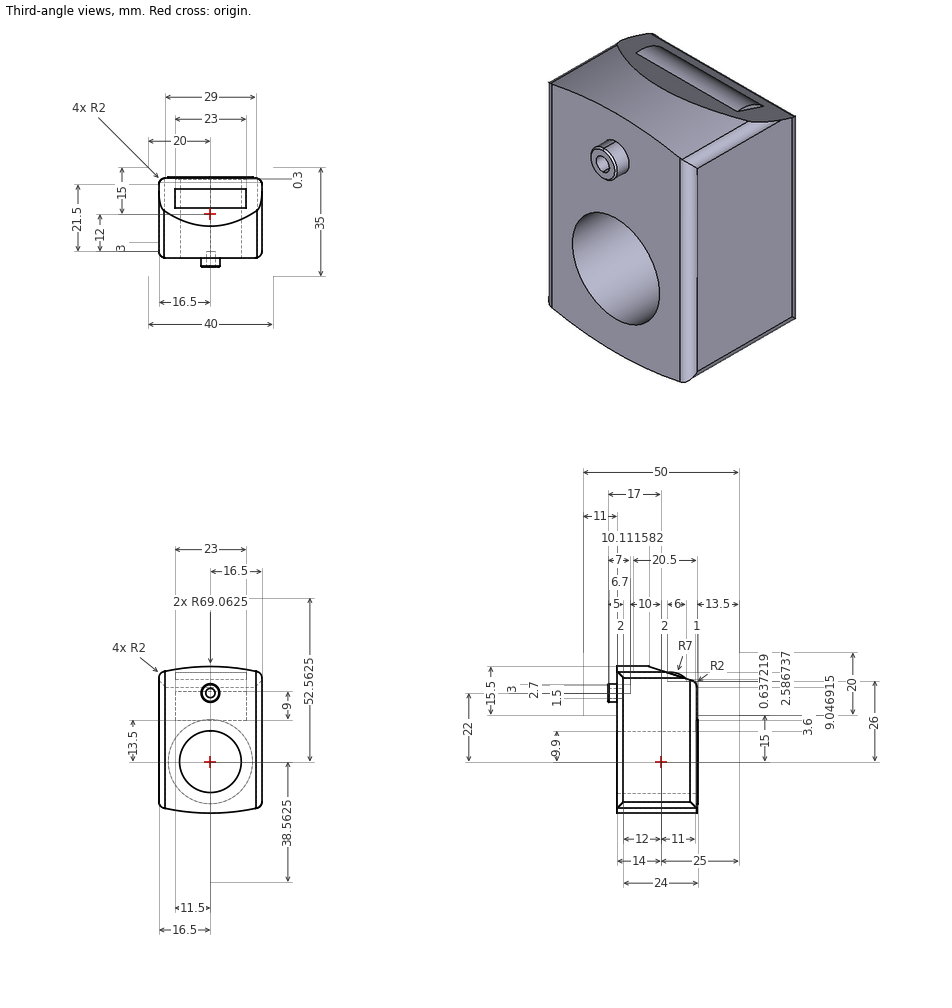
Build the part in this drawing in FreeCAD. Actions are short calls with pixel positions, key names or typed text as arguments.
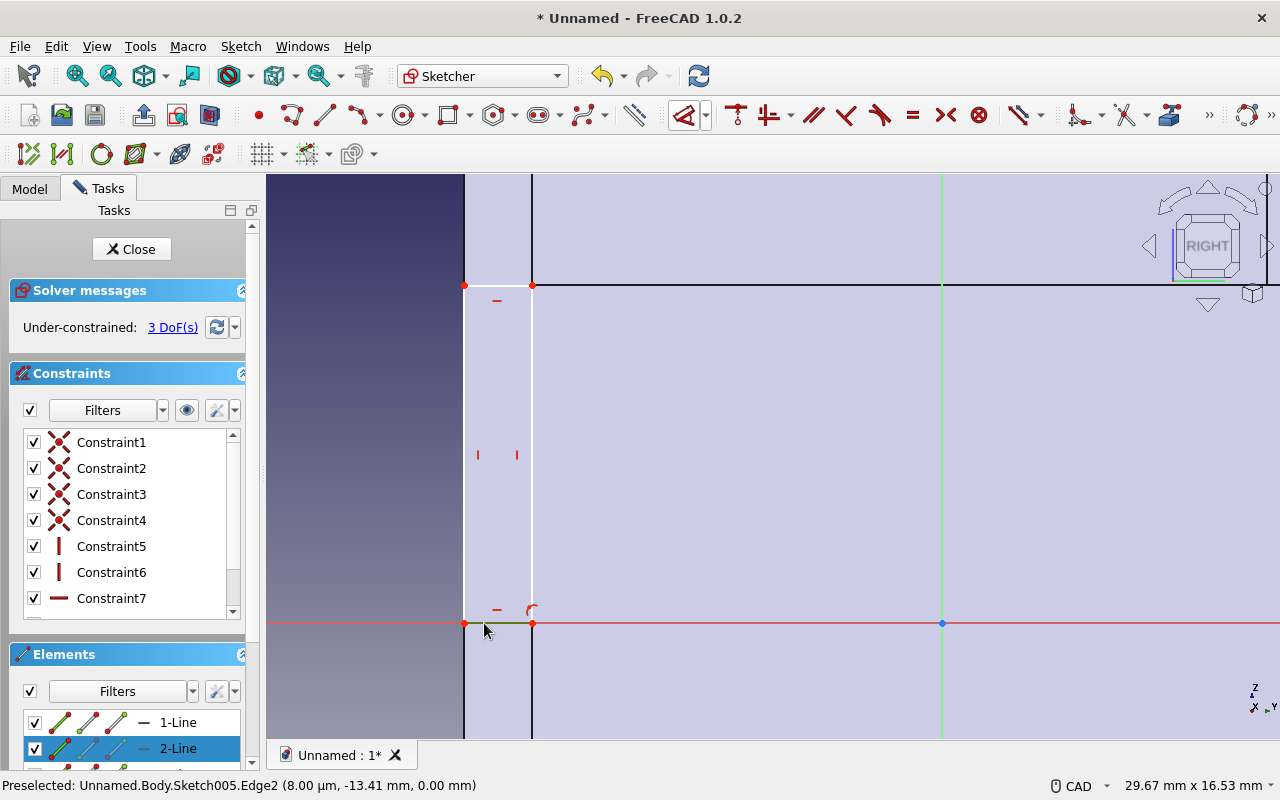
key(l)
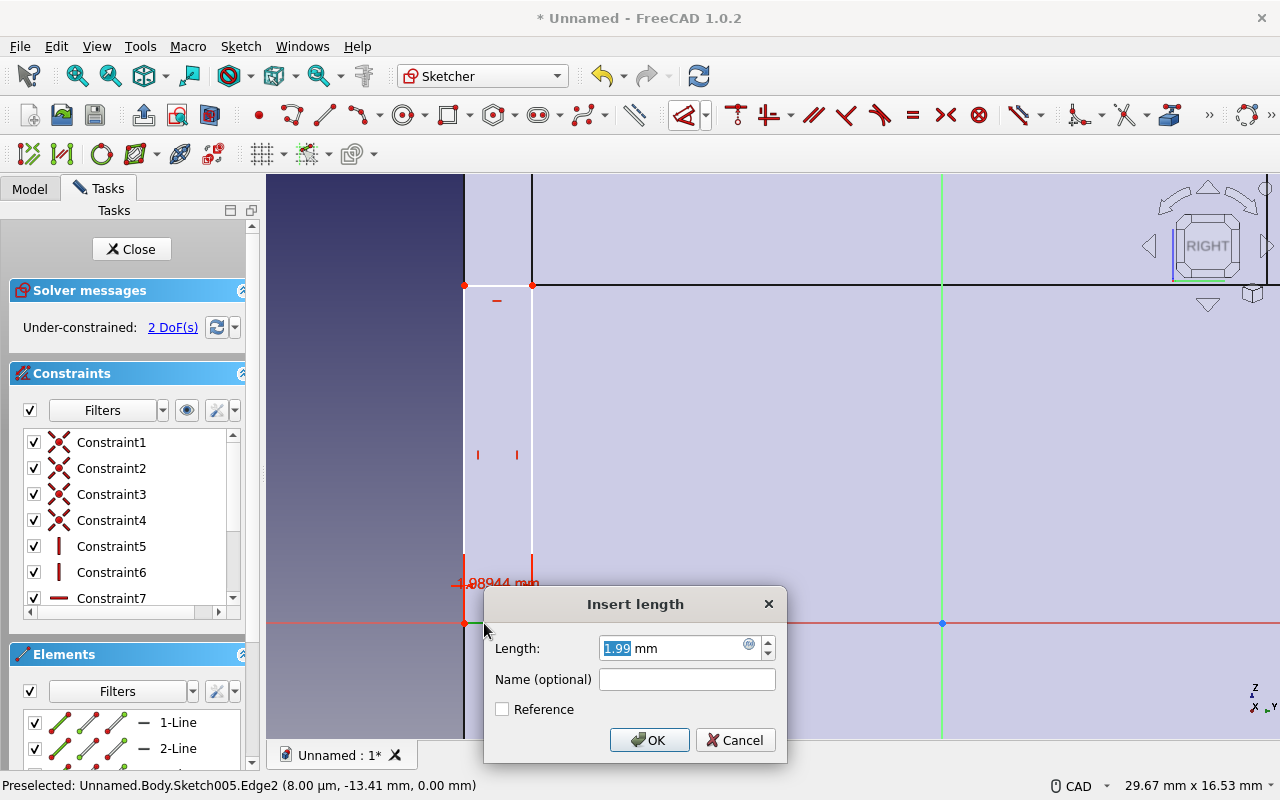
text(2)
key(Return)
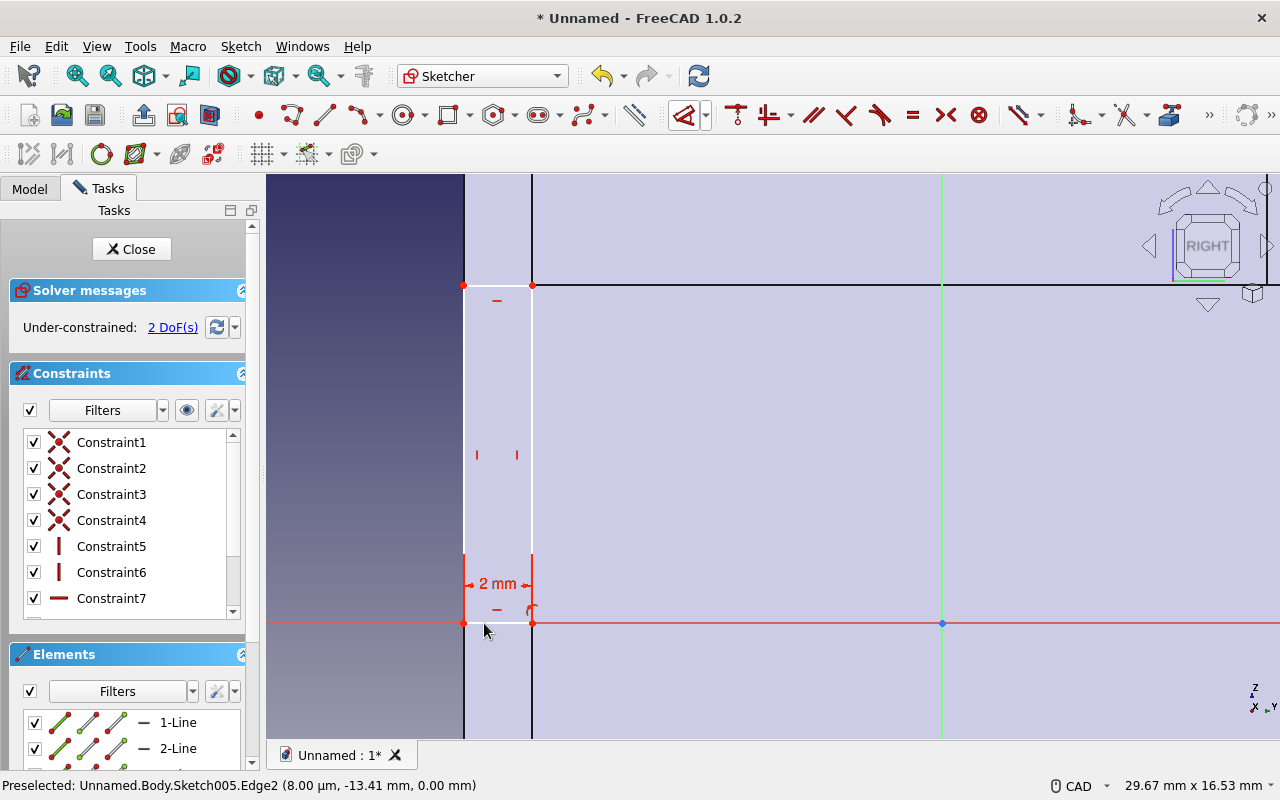
click(464, 387)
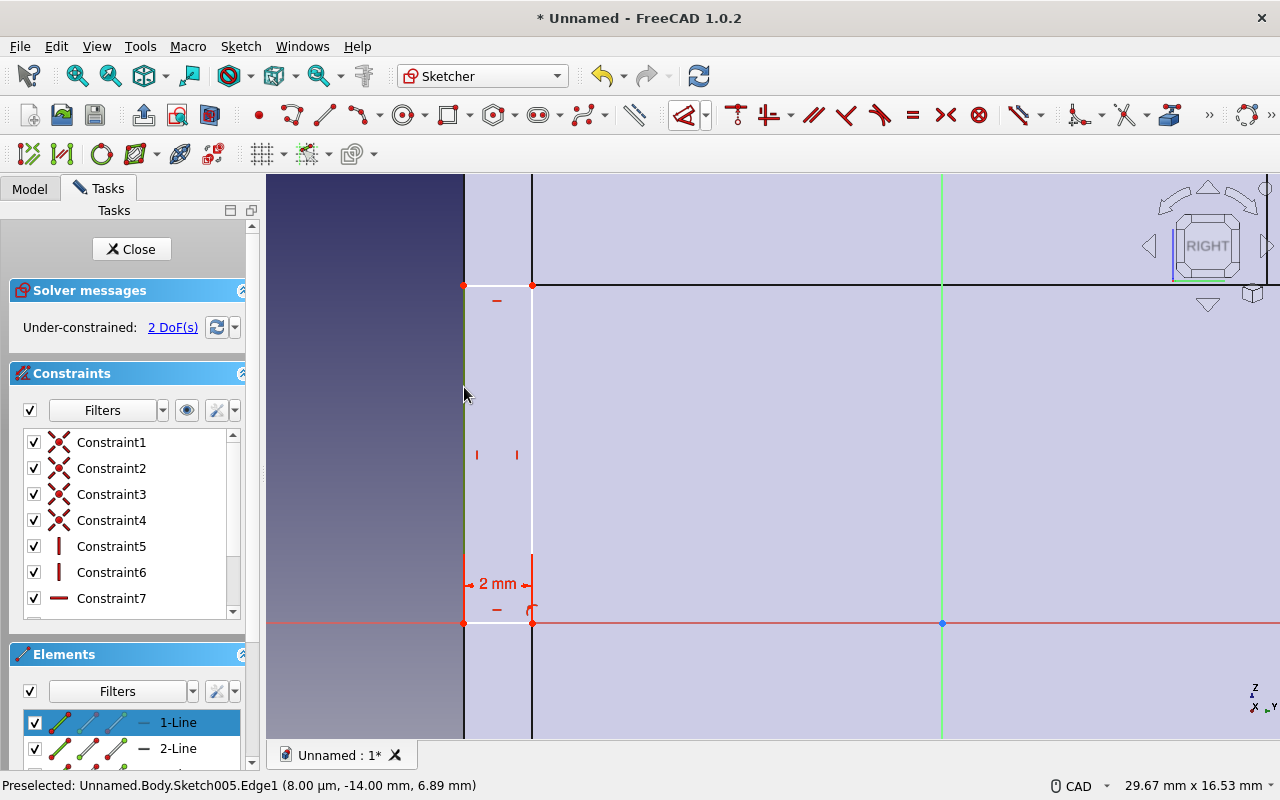
key(i)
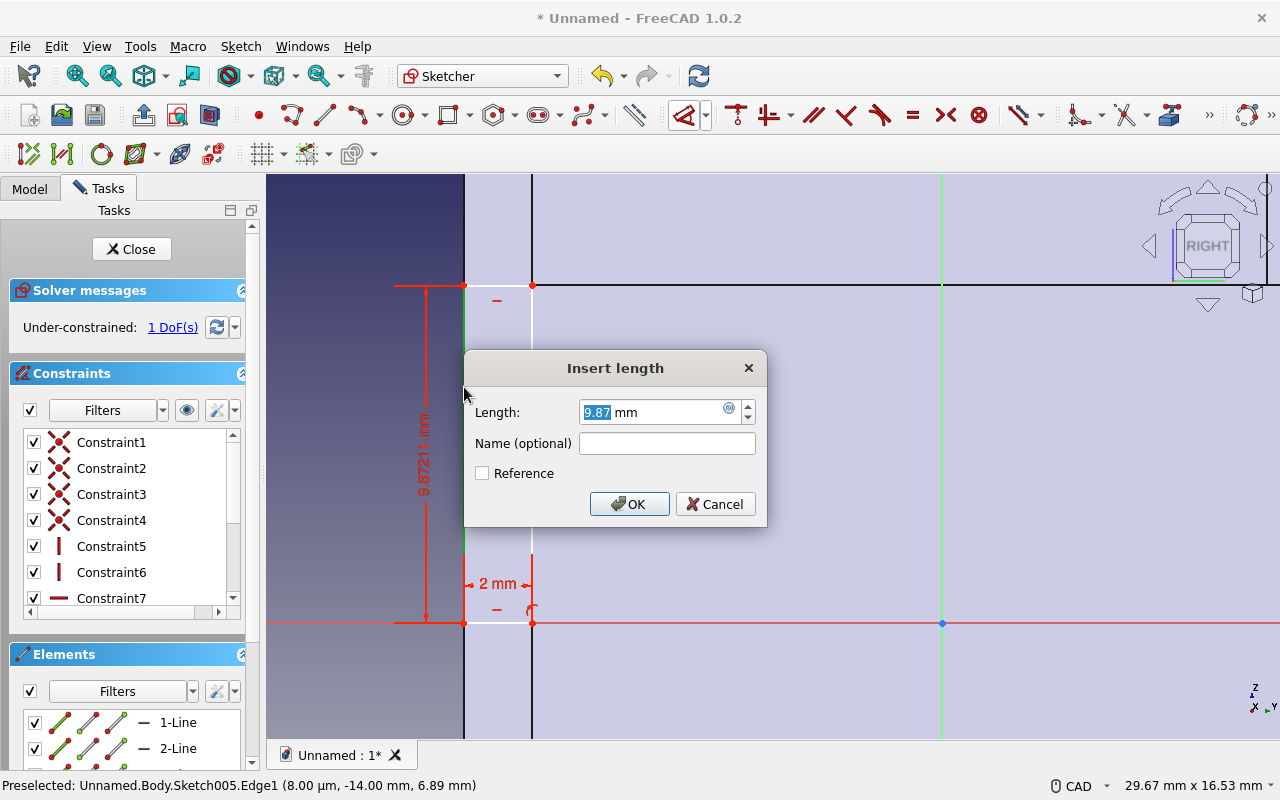
text(9.9)
key(Return)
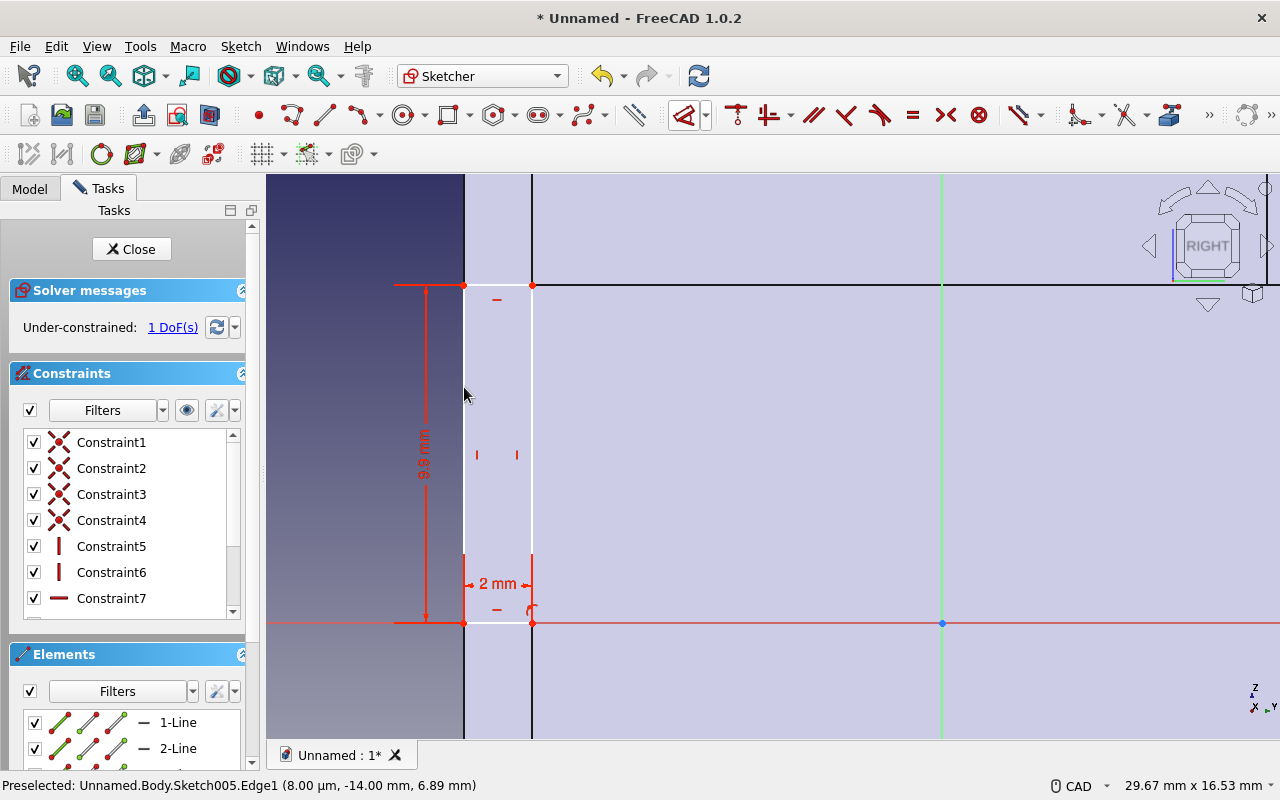
click(464, 285)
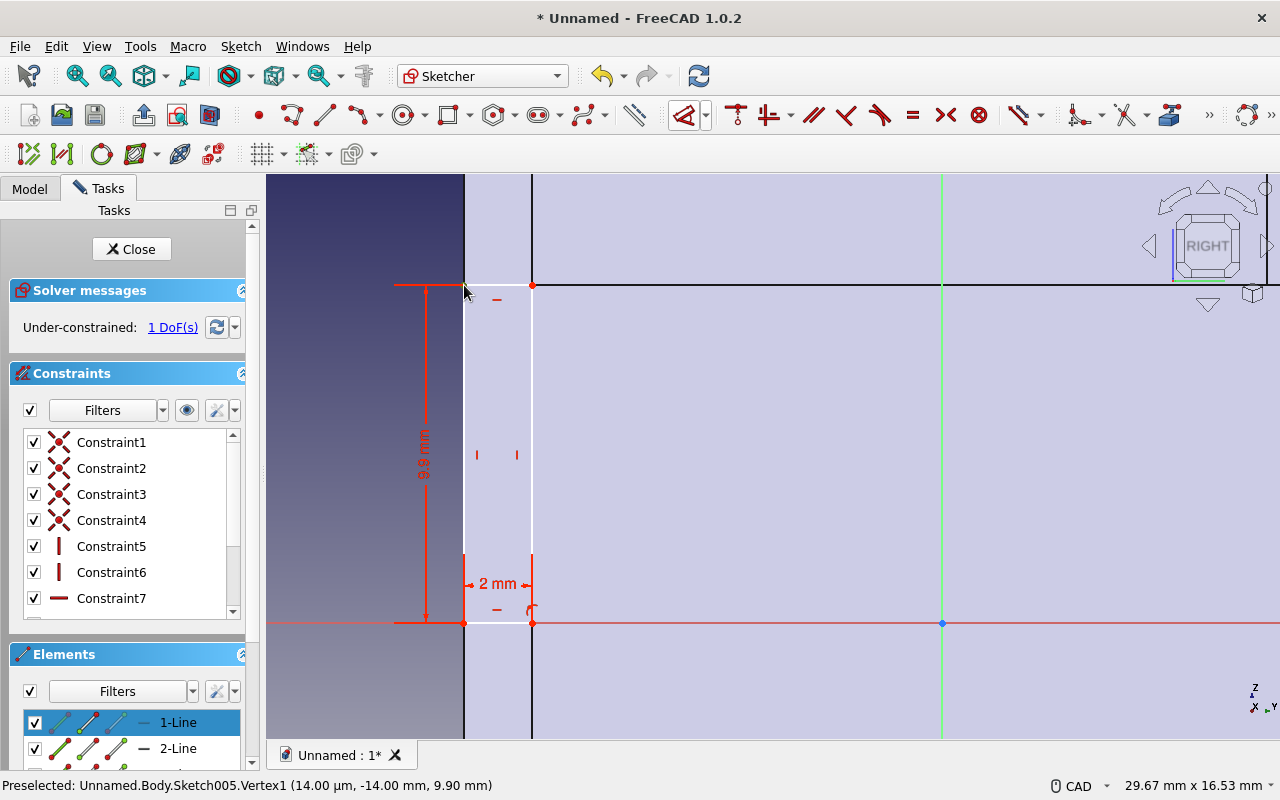
key(l)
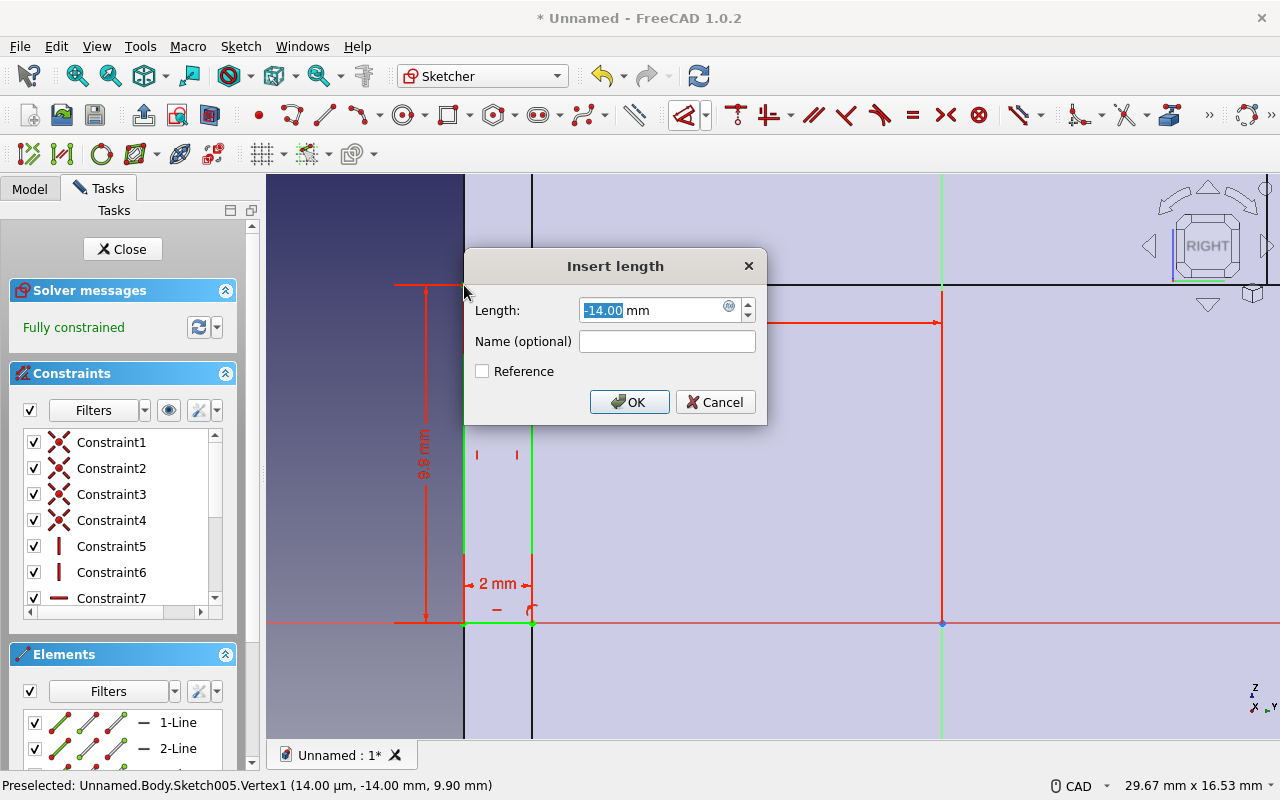
text(-14)
key(Return)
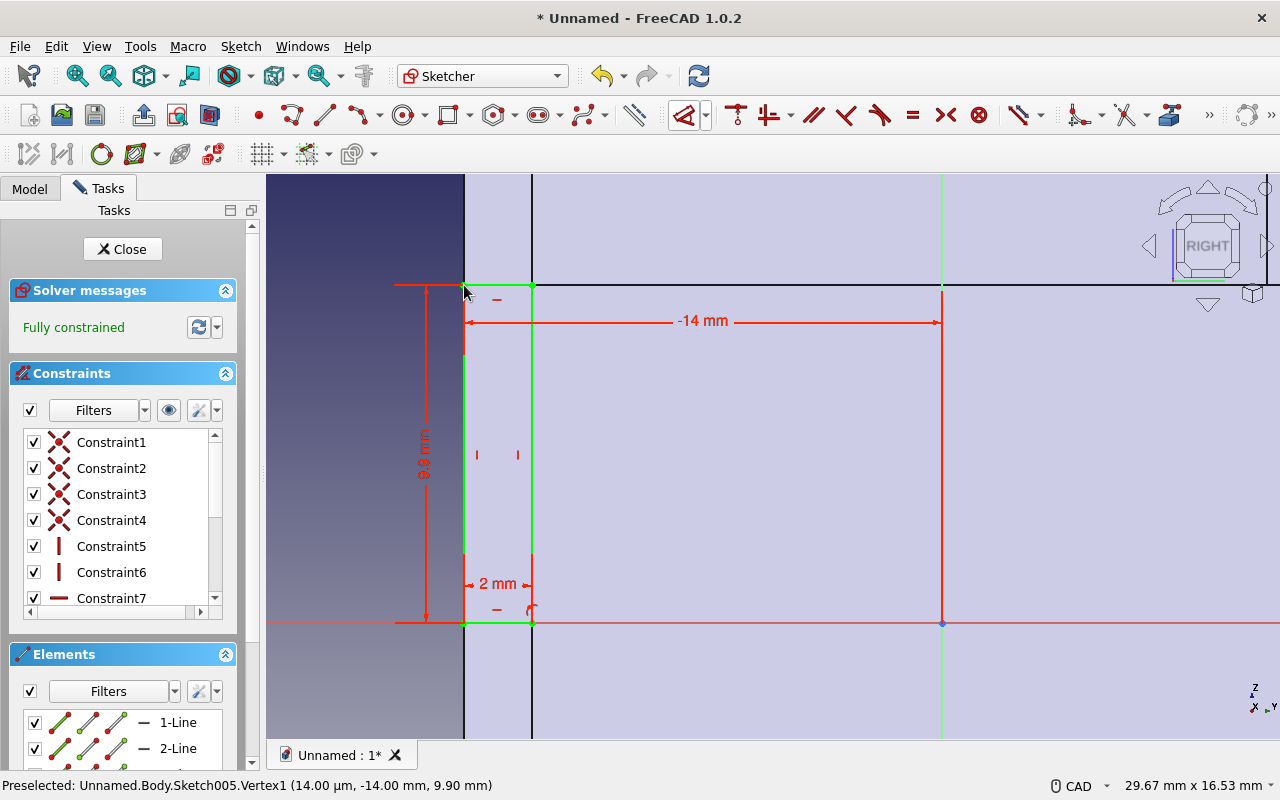
click(123, 249)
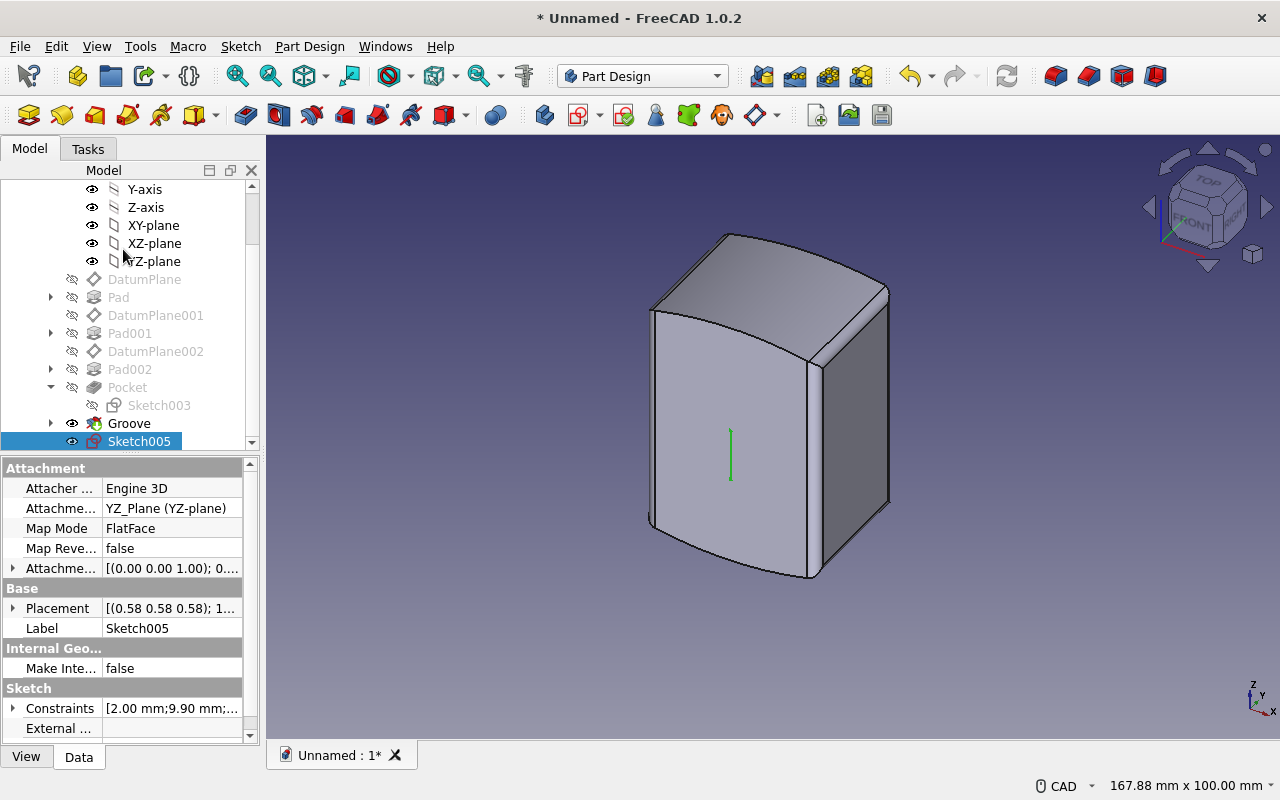
click(312, 116)